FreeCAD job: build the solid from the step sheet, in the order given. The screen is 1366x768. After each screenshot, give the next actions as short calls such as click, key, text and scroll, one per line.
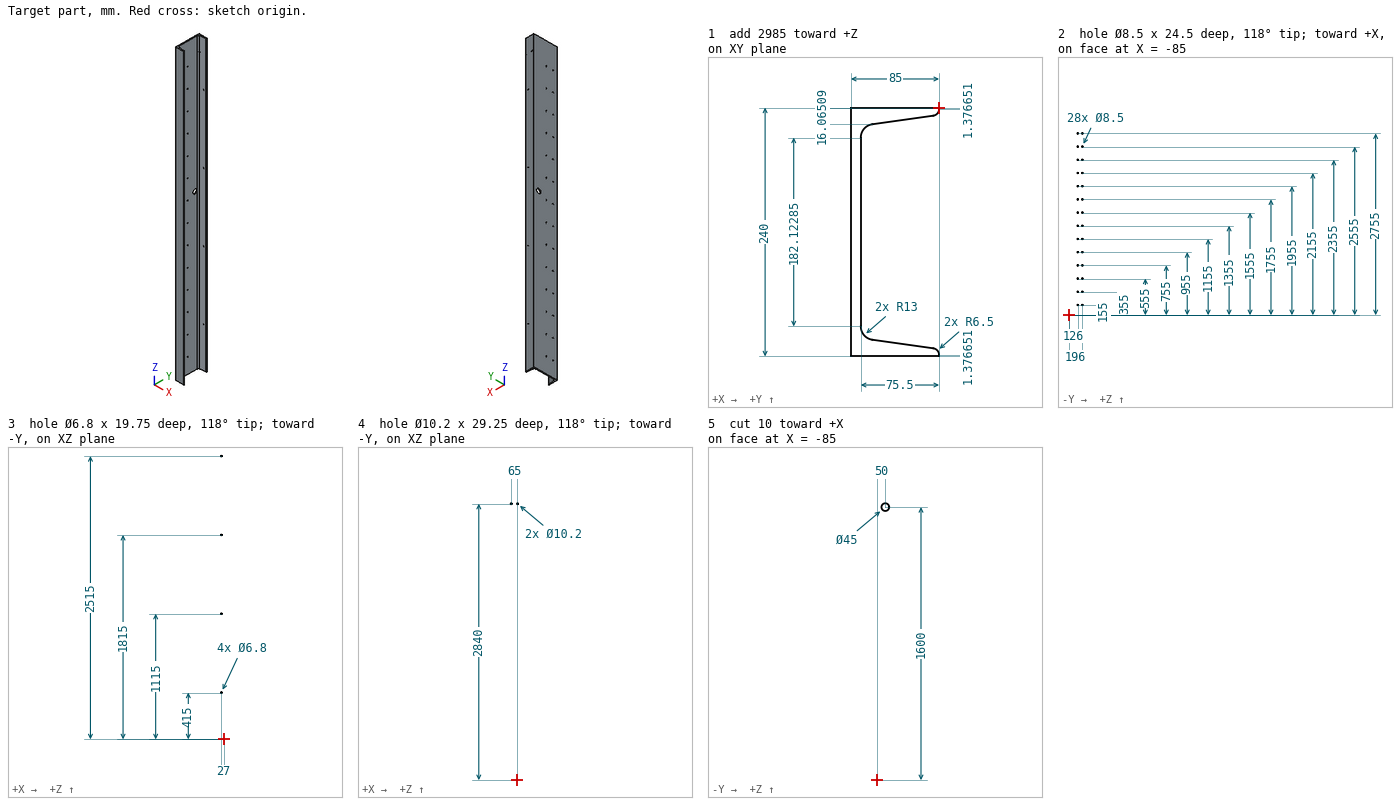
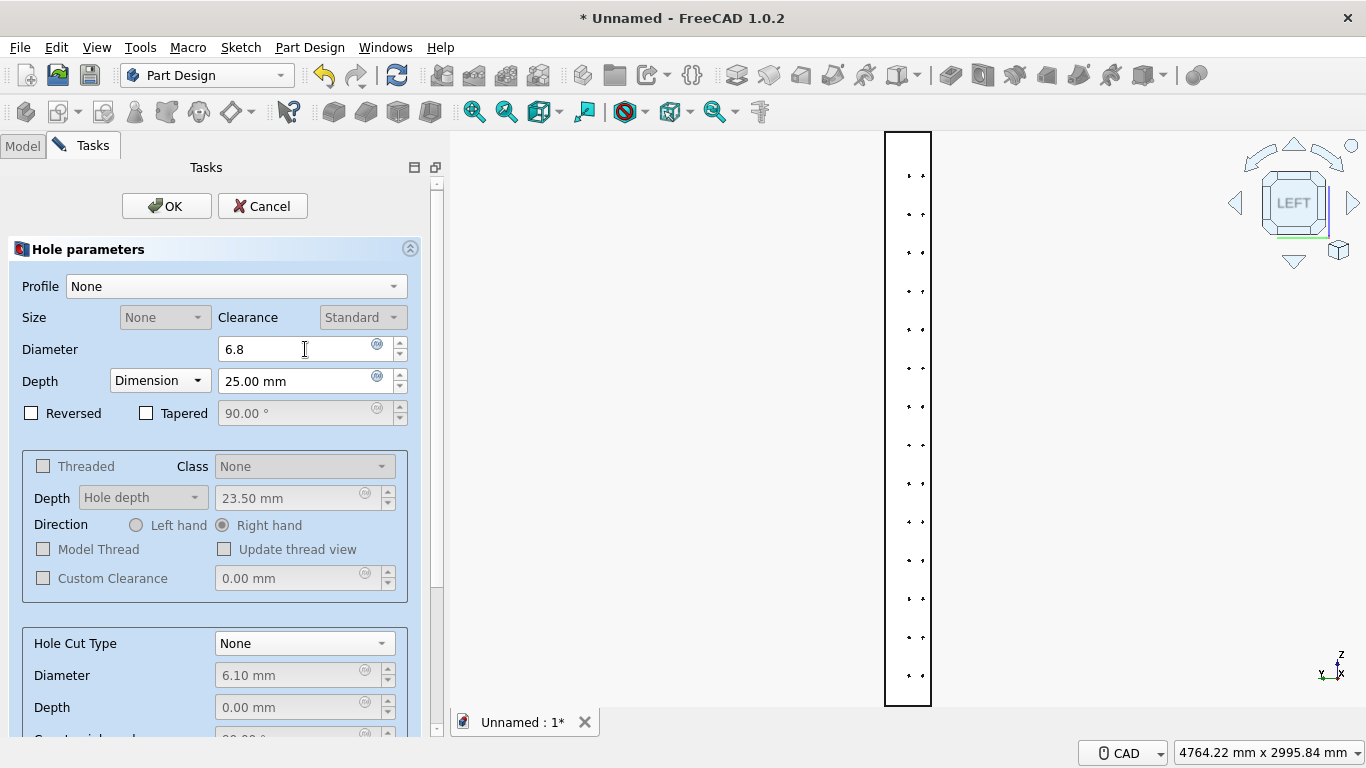
triple_click(305, 381)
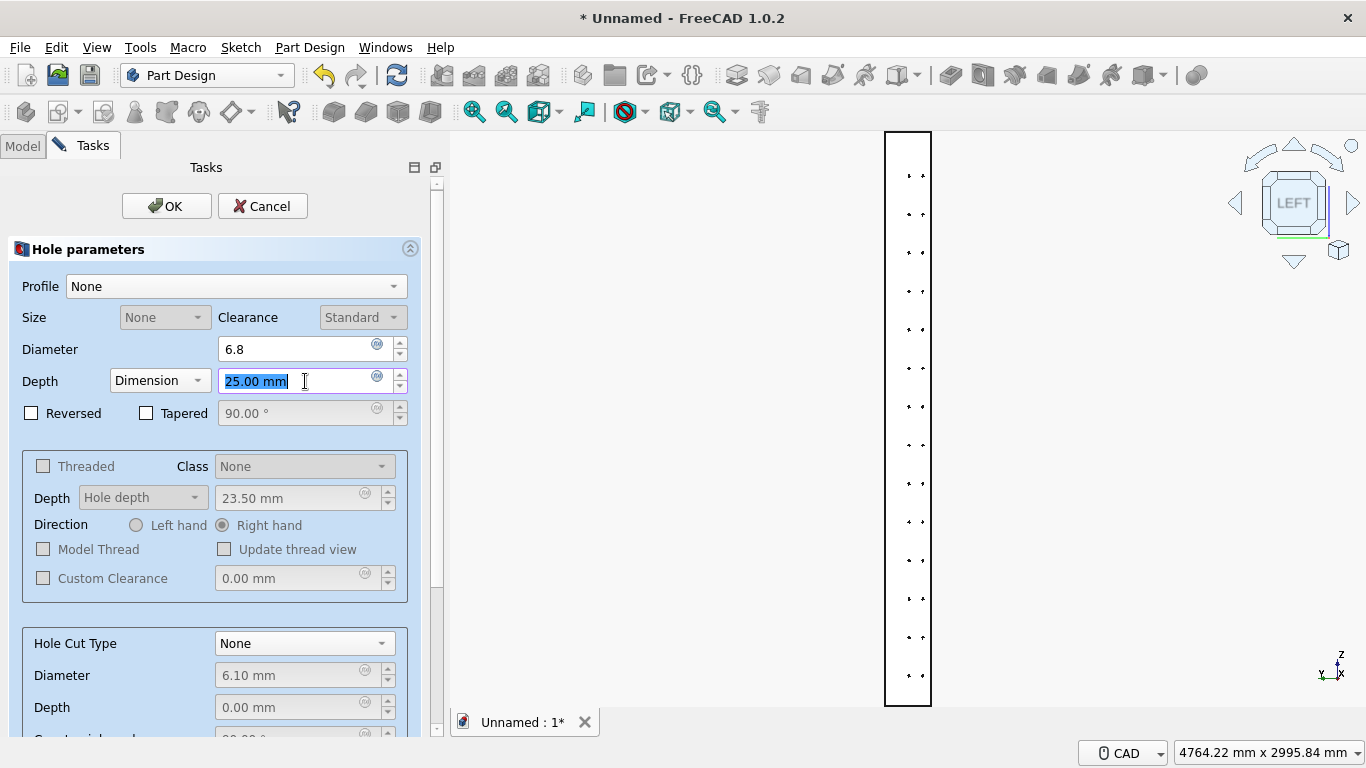
text(19.75)
key(Tab)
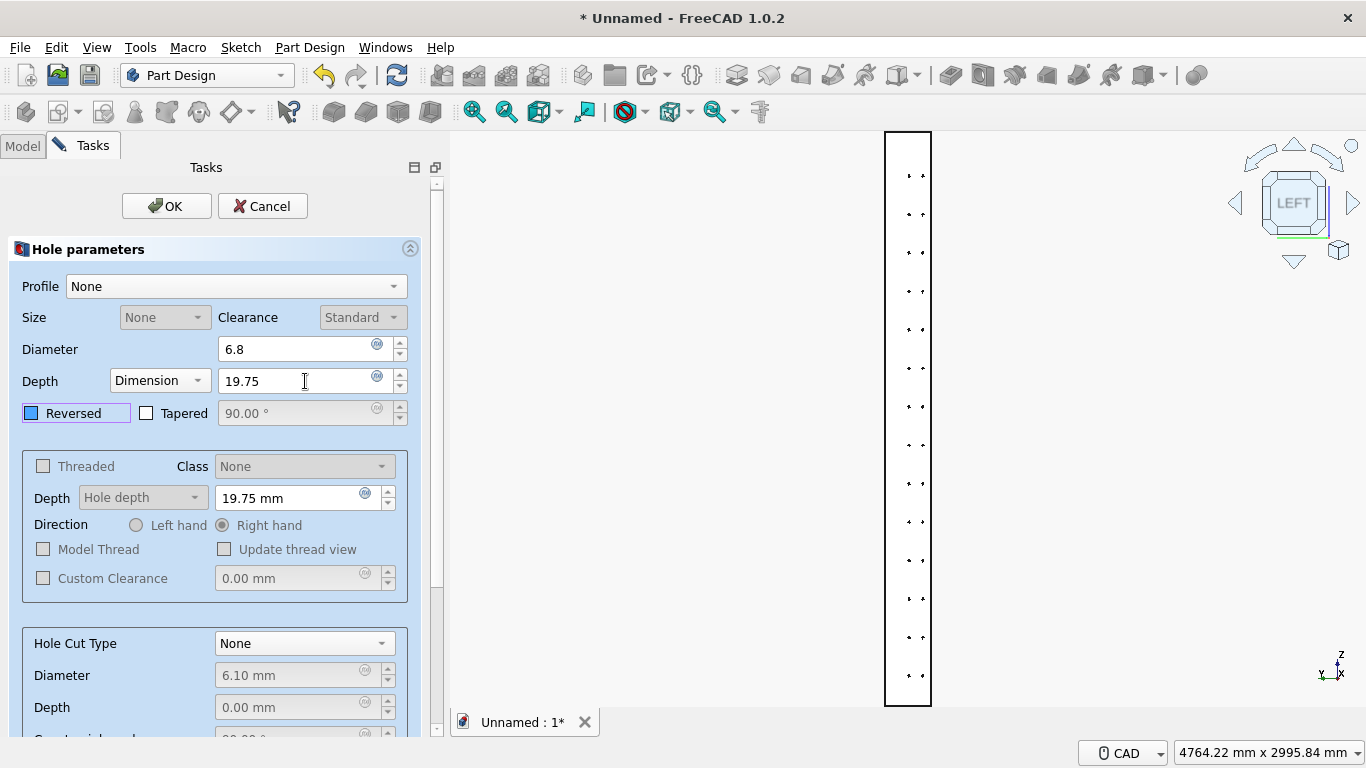
click(30, 413)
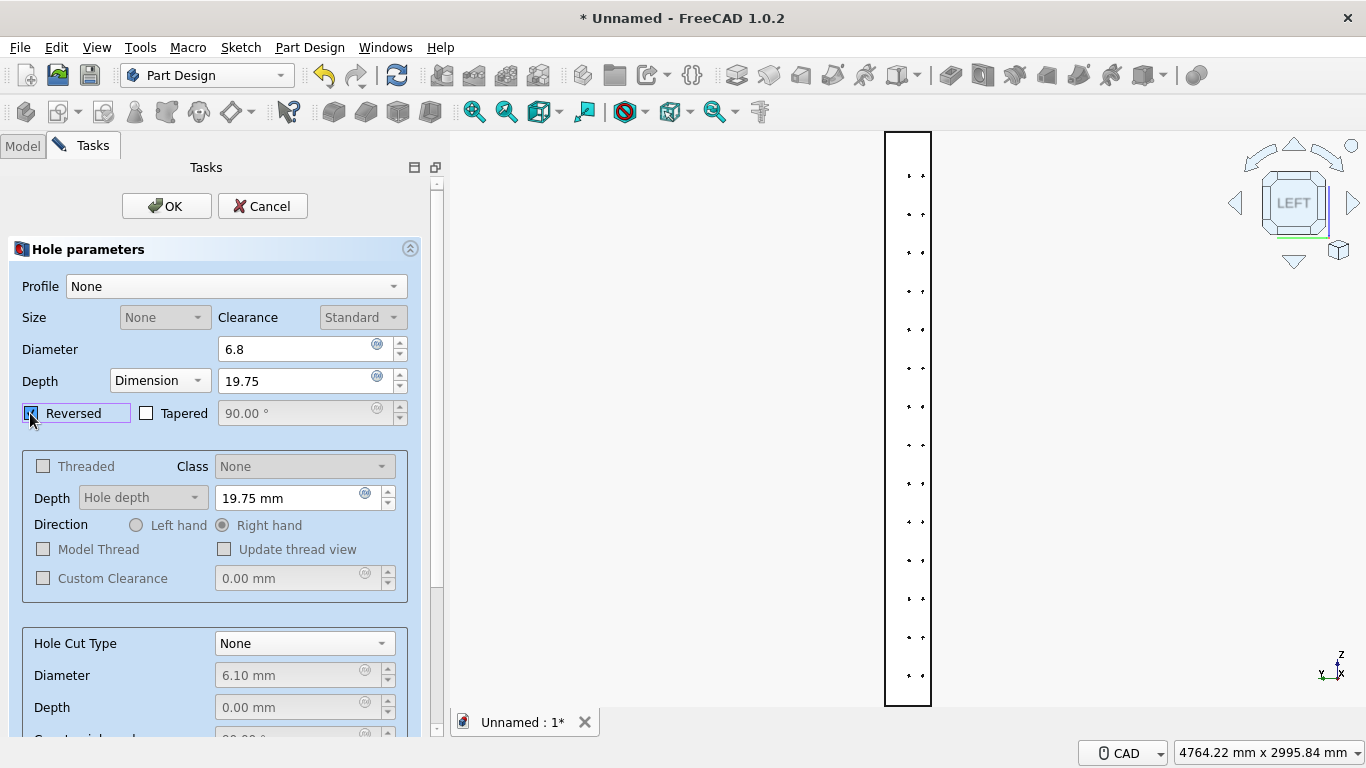
click(167, 206)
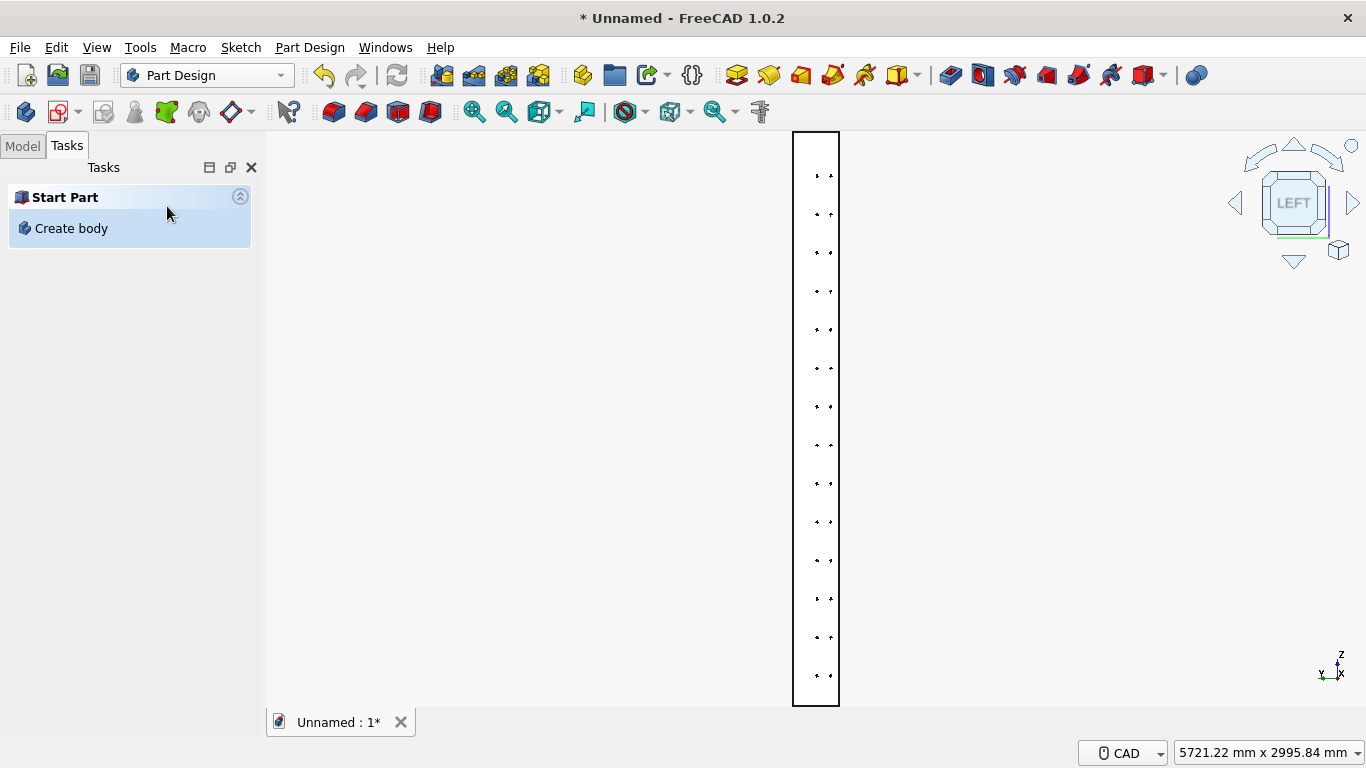
click(58, 112)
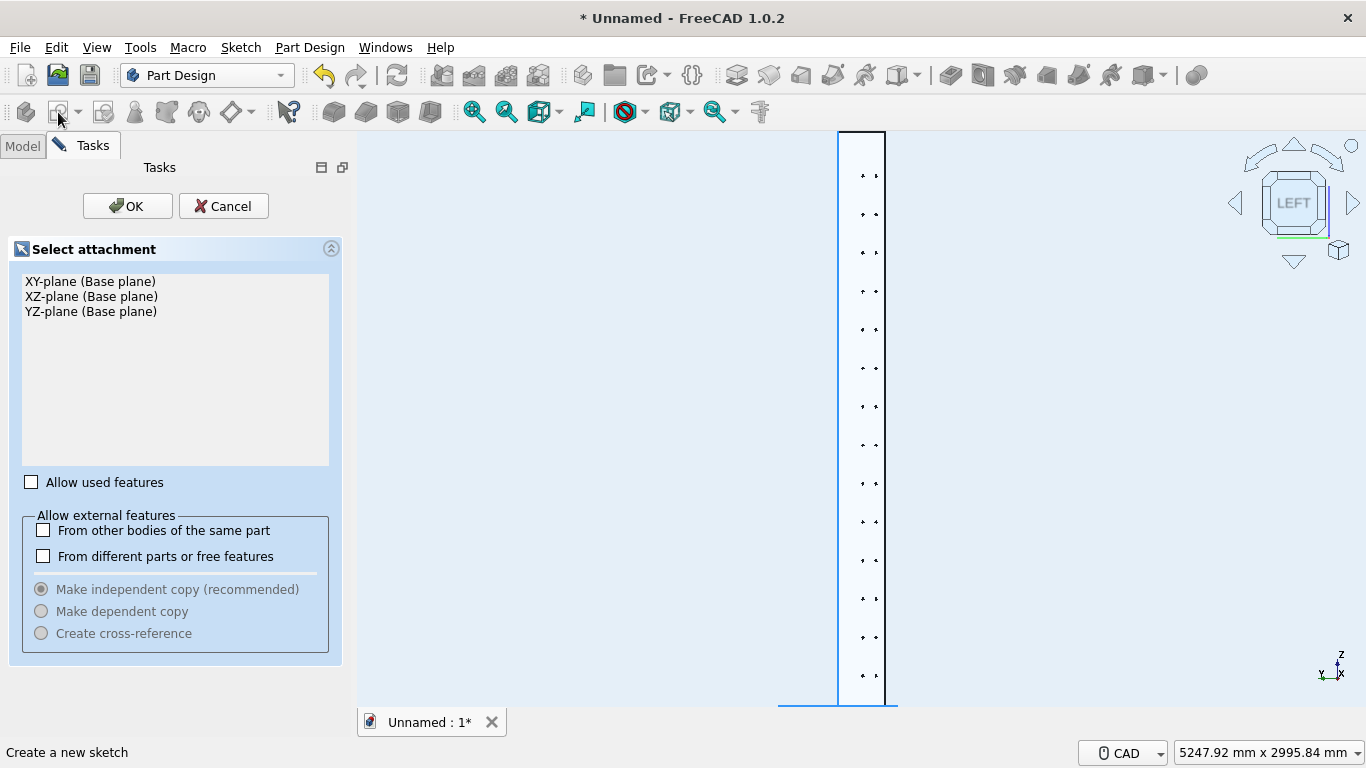
click(82, 296)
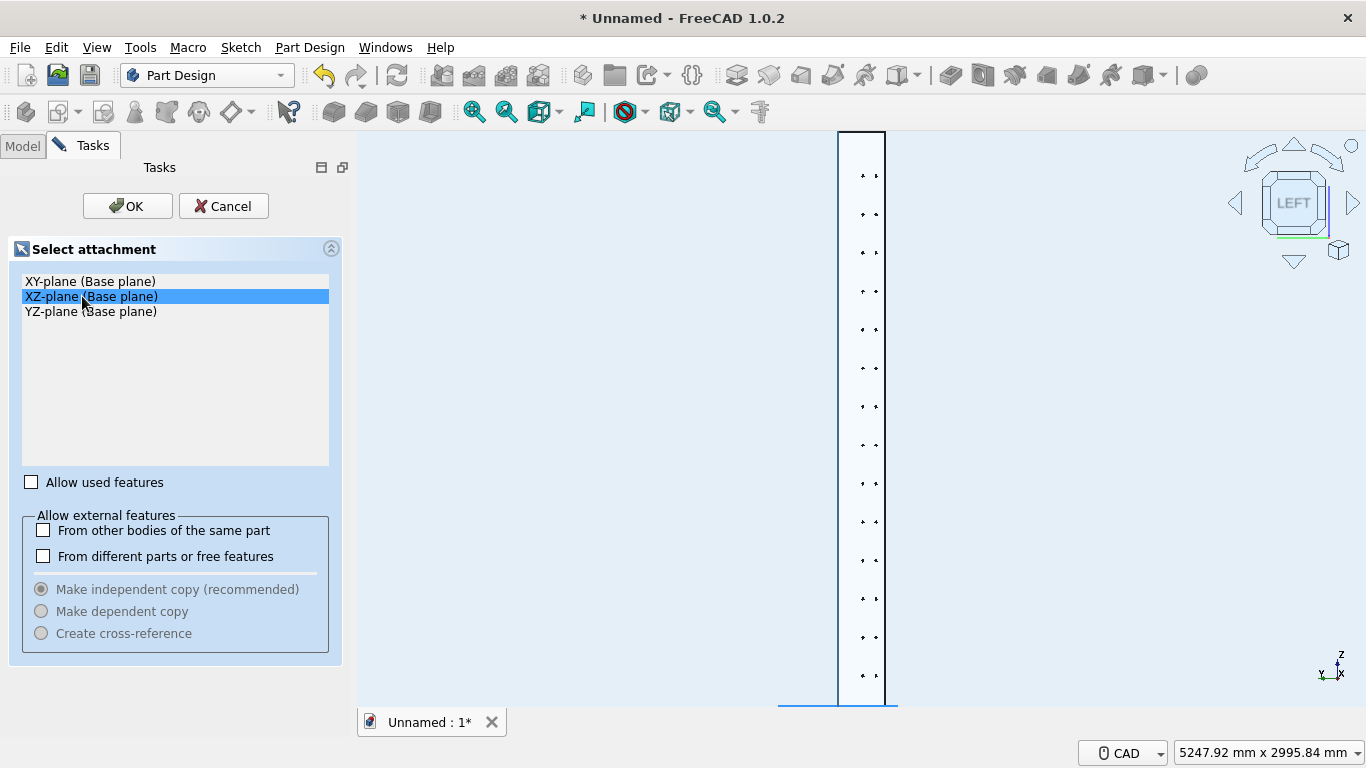
click(128, 206)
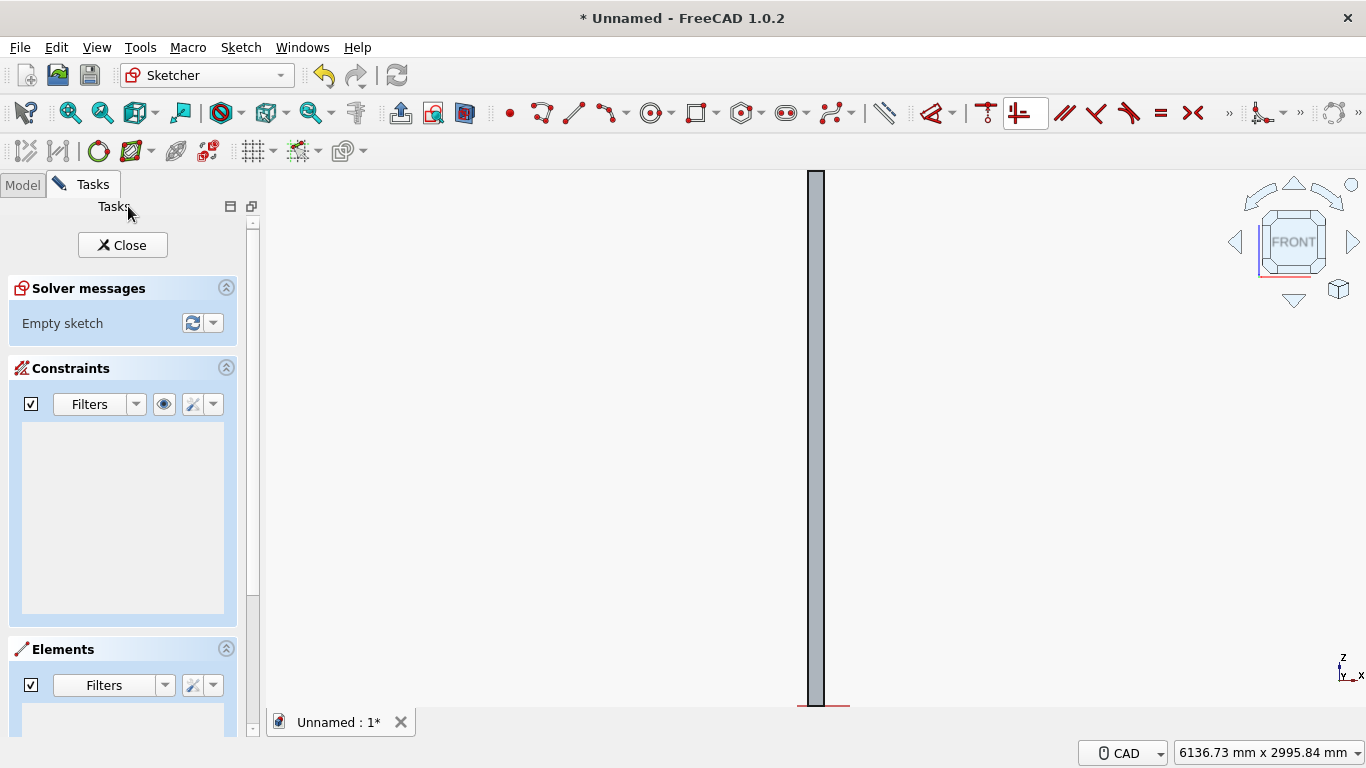
click(466, 114)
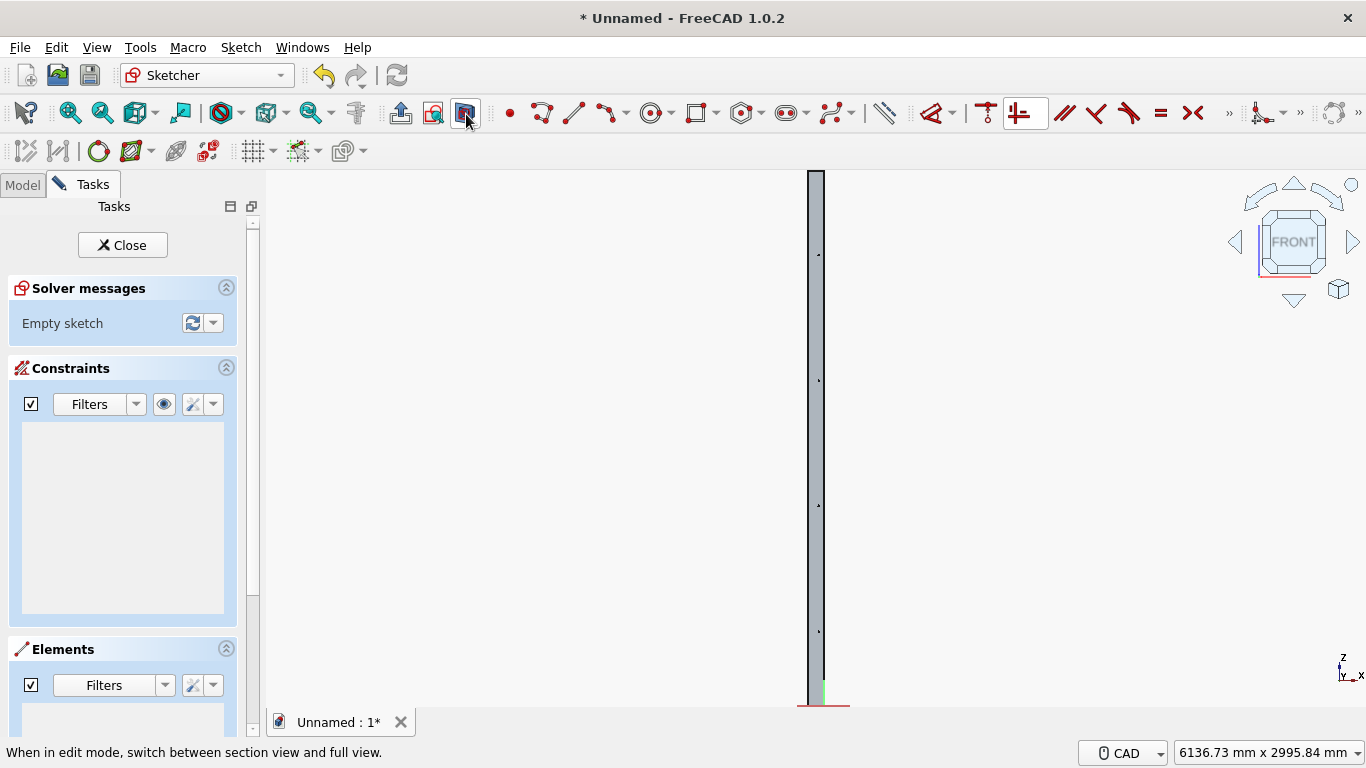
scroll(748, 438, down, 5)